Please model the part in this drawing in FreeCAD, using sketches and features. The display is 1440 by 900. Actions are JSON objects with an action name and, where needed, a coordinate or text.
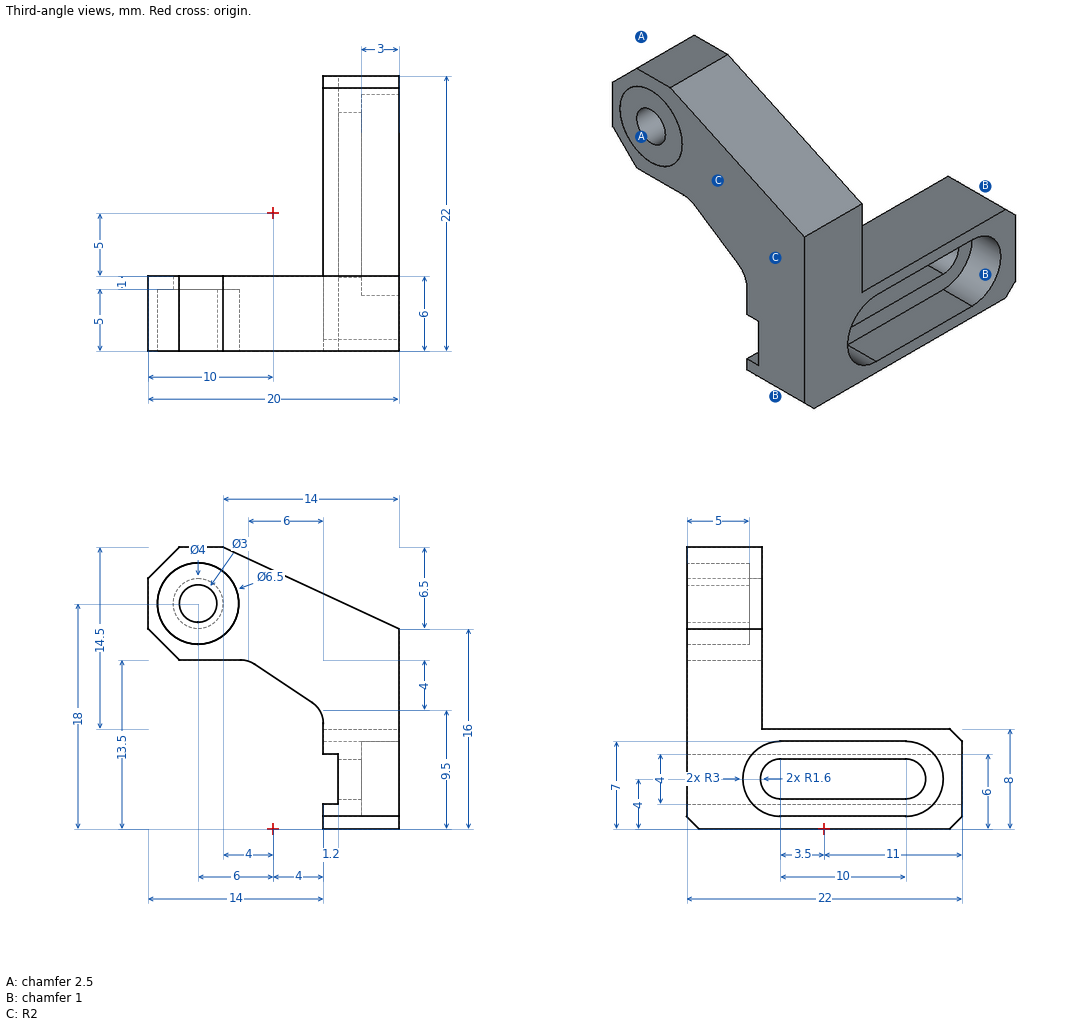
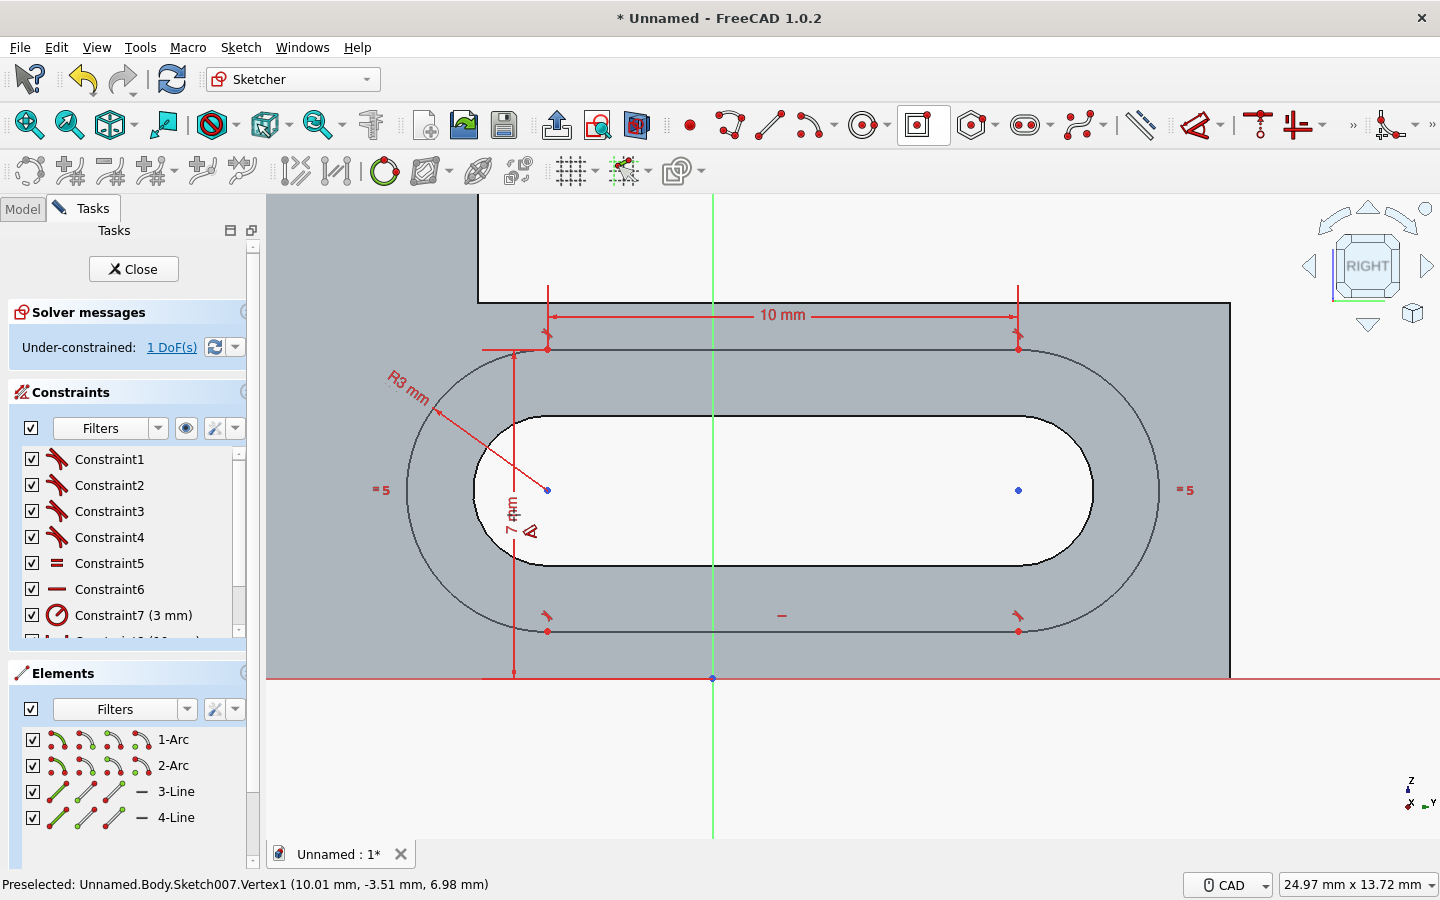
{"action": "left_click", "coordinate": [548, 350]}
{"action": "left_click", "coordinate": [630, 713]}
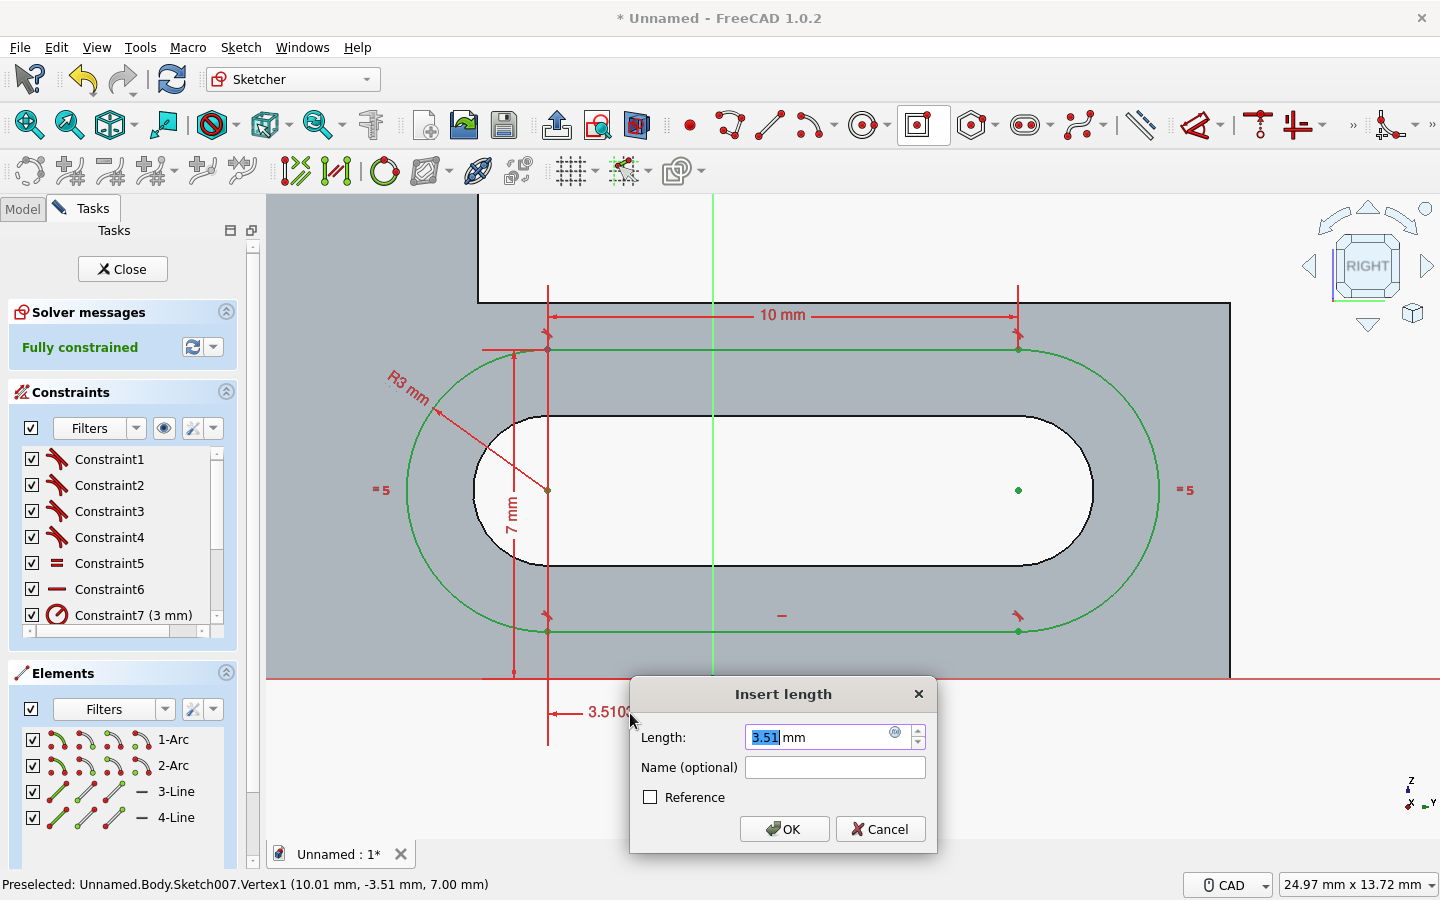
{"action": "type", "text": "3.5"}
{"action": "key", "text": "Return"}
{"action": "key", "text": "Escape"}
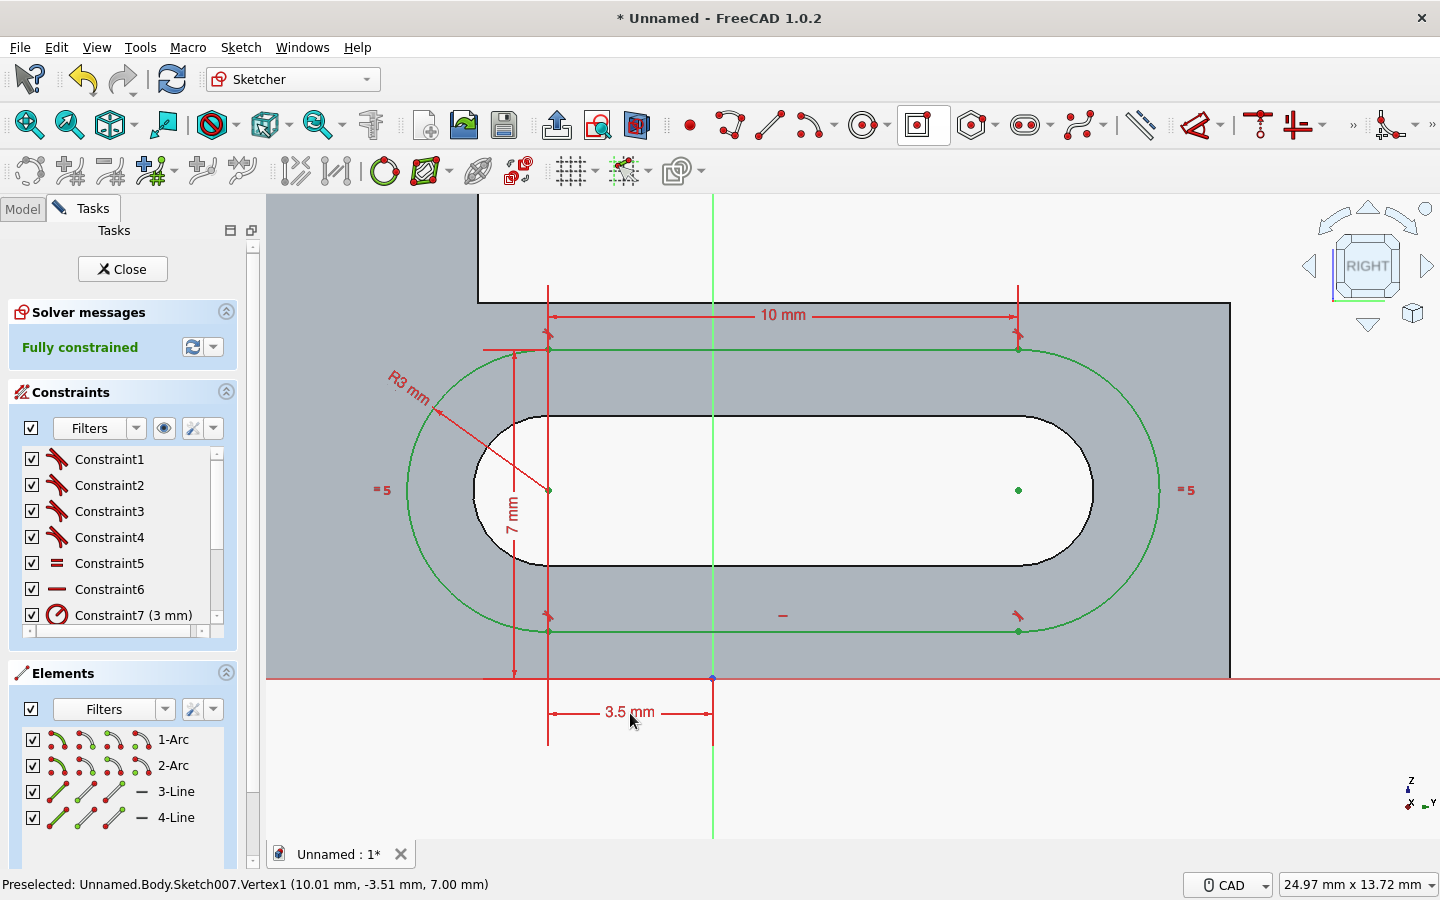
{"action": "left_click", "coordinate": [123, 269]}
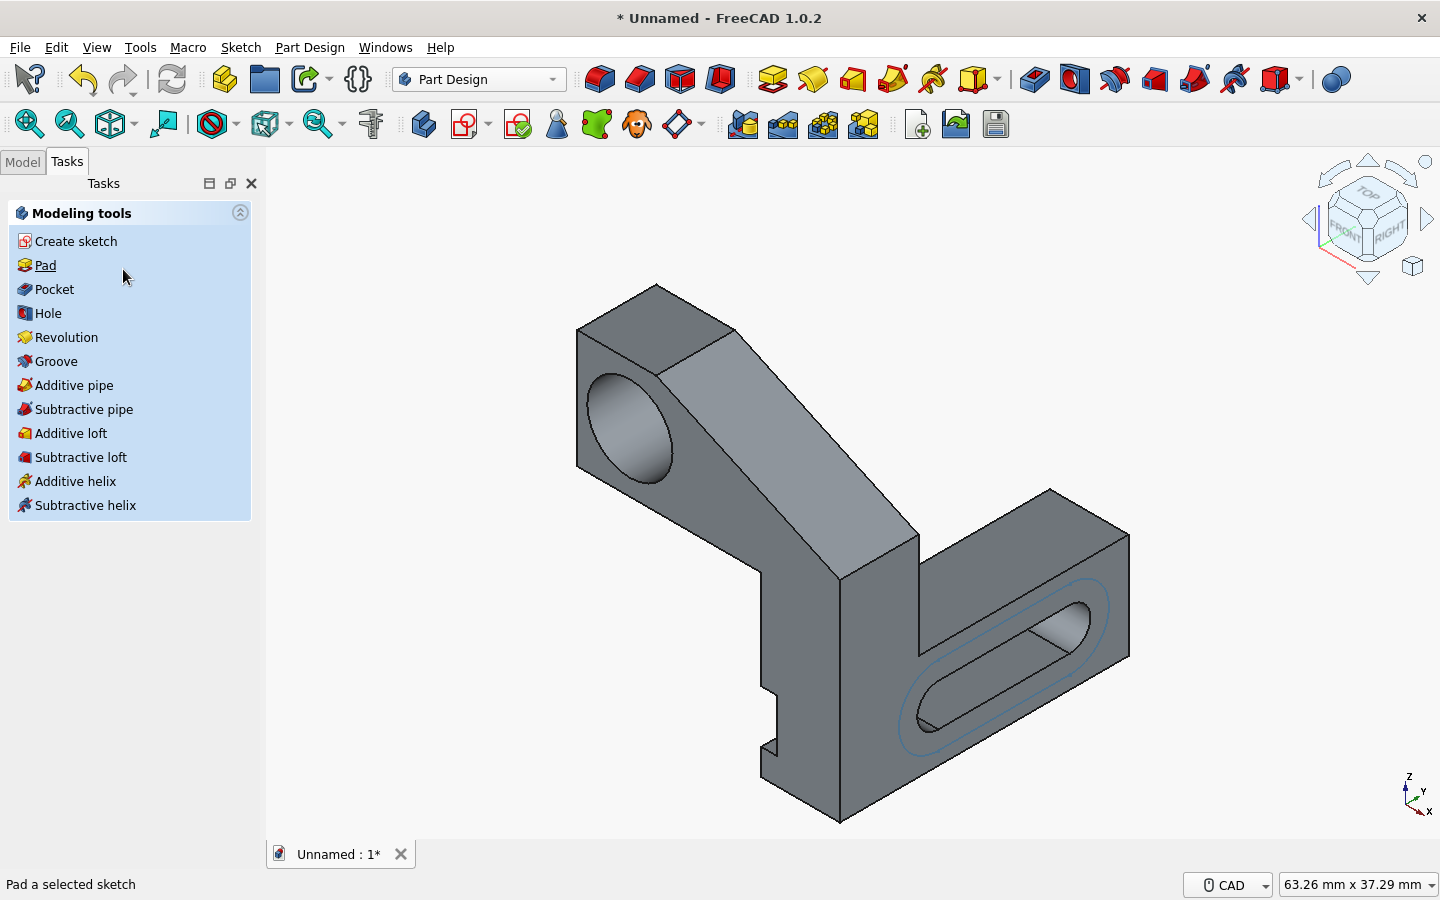
{"action": "left_click", "coordinate": [1036, 80]}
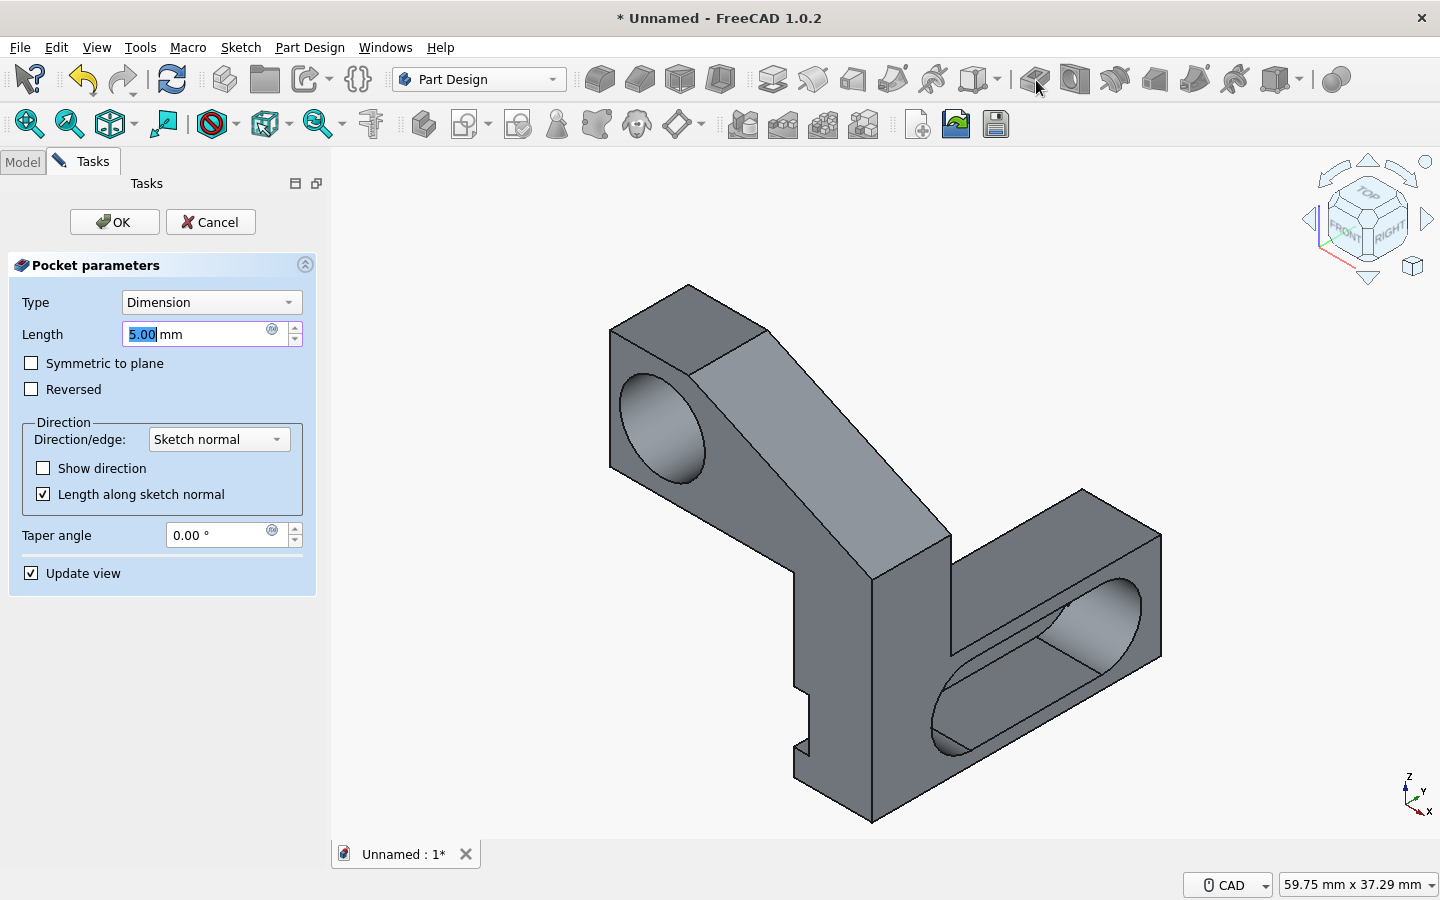
{"action": "type", "text": "3"}
{"action": "key", "text": "Tab"}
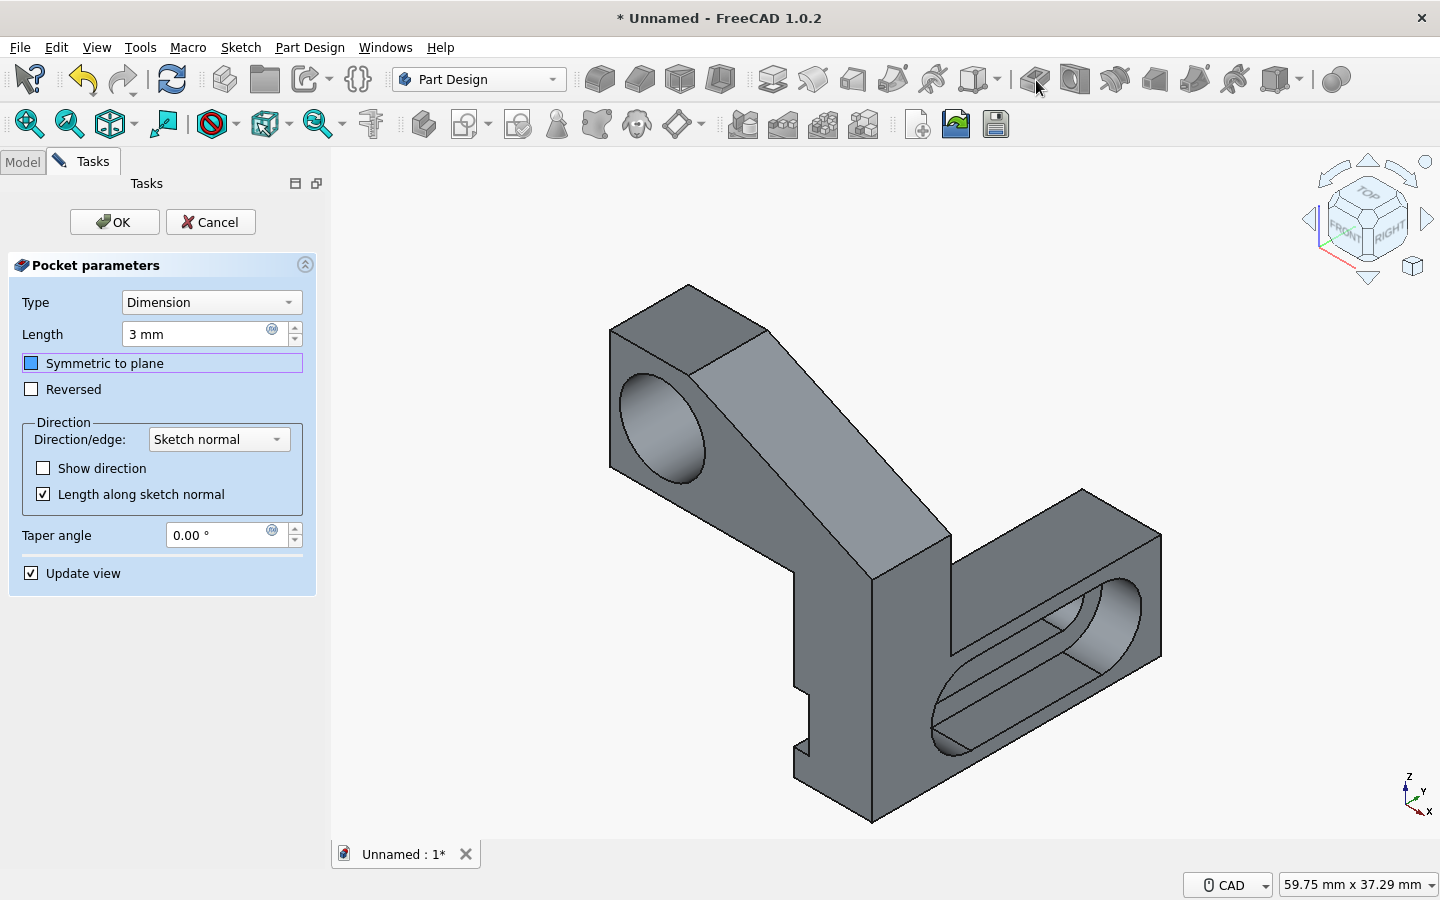
{"action": "left_click", "coordinate": [115, 222]}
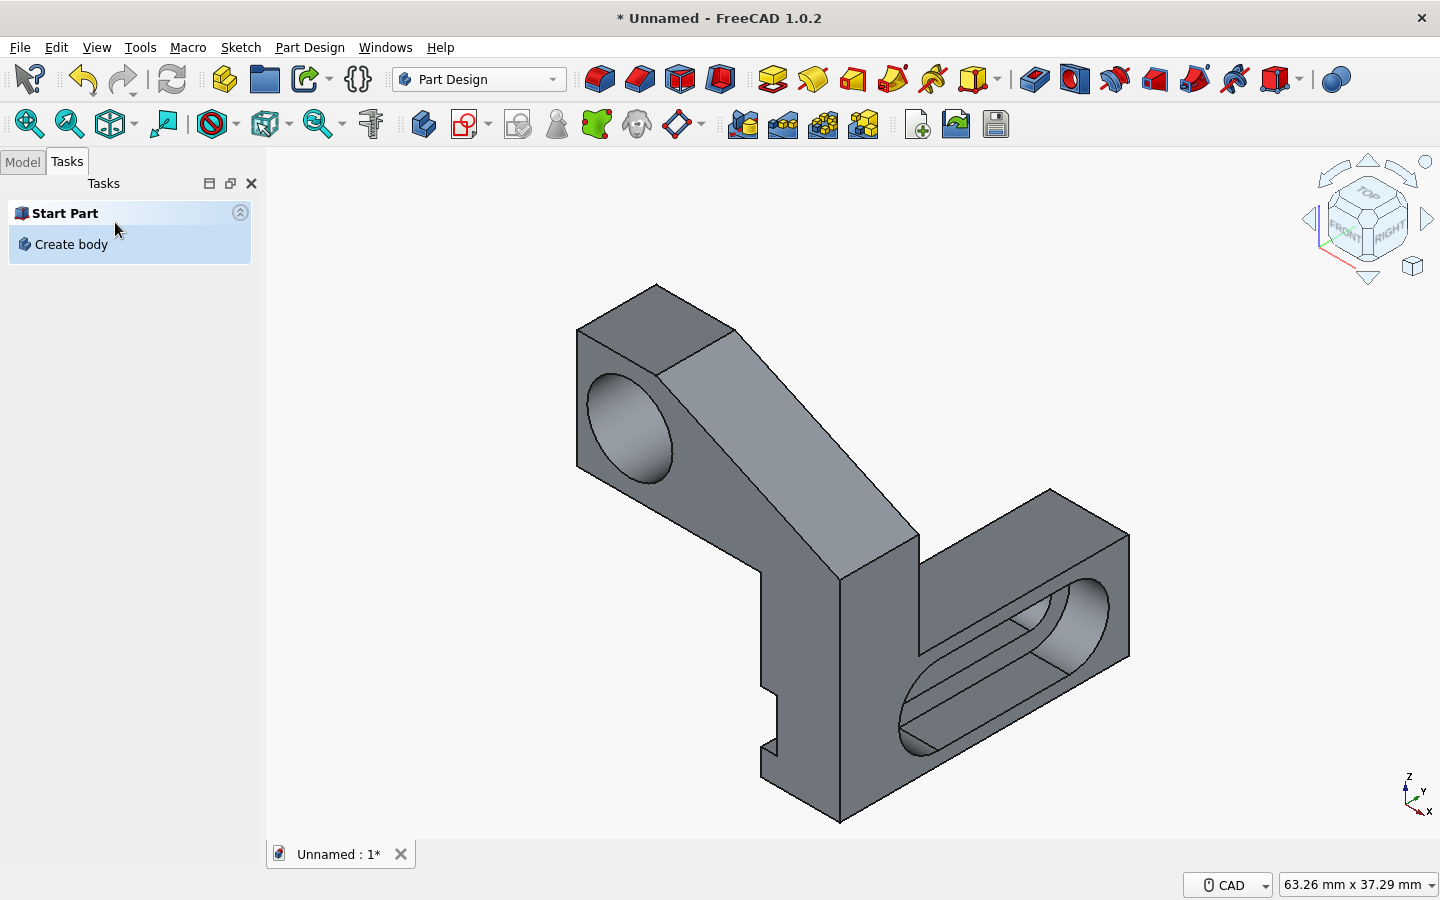
{"action": "key", "text": "2"}